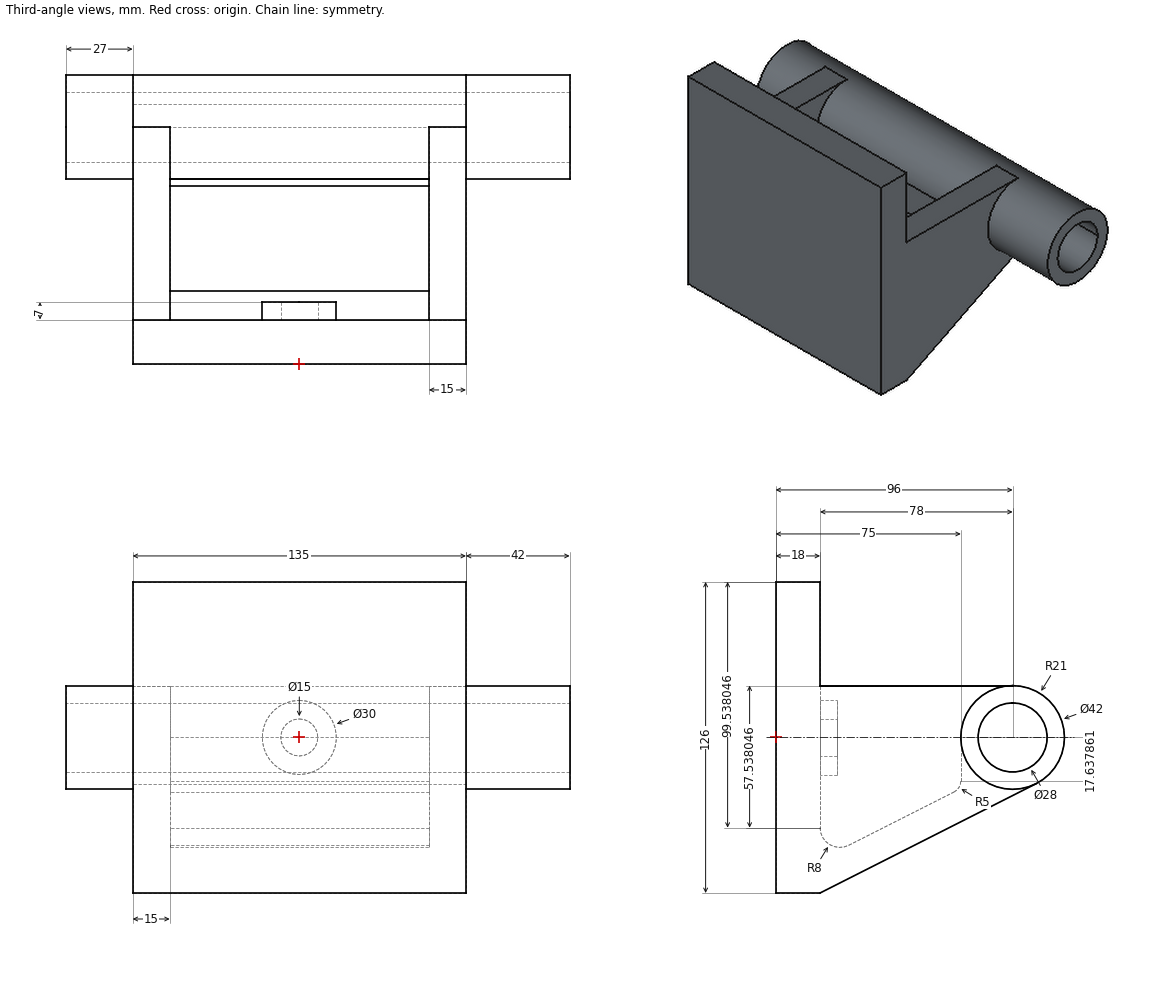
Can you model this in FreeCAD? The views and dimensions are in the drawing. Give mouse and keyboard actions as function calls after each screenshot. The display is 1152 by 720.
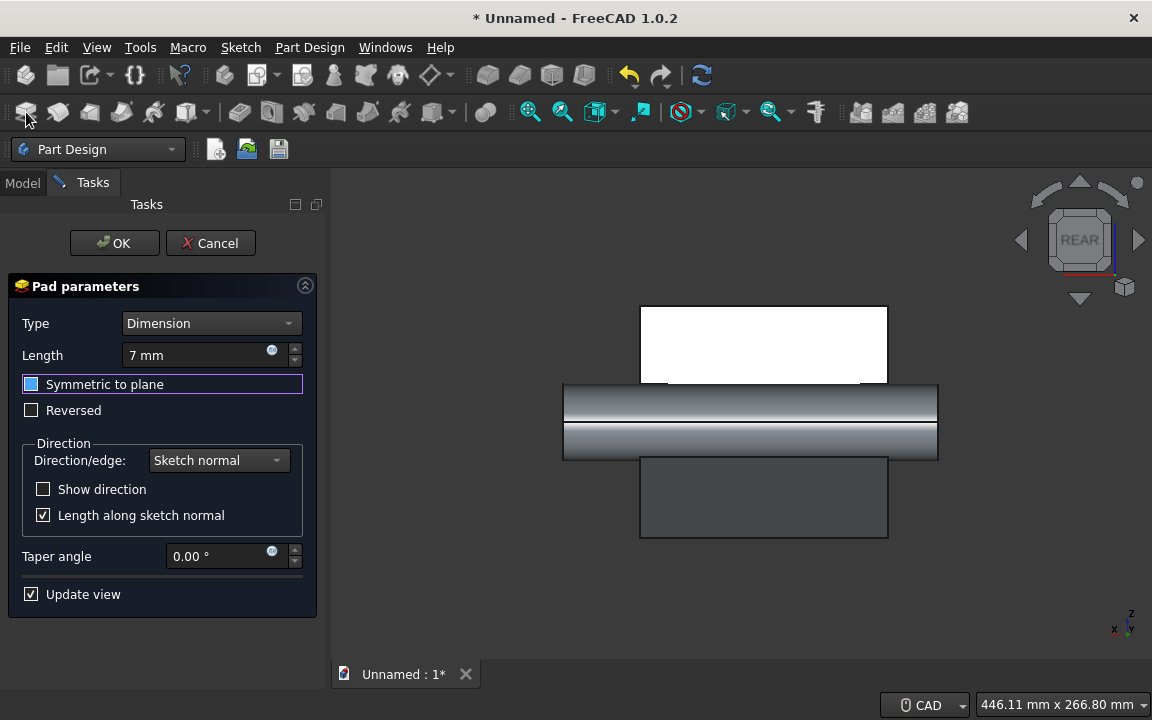
click(115, 243)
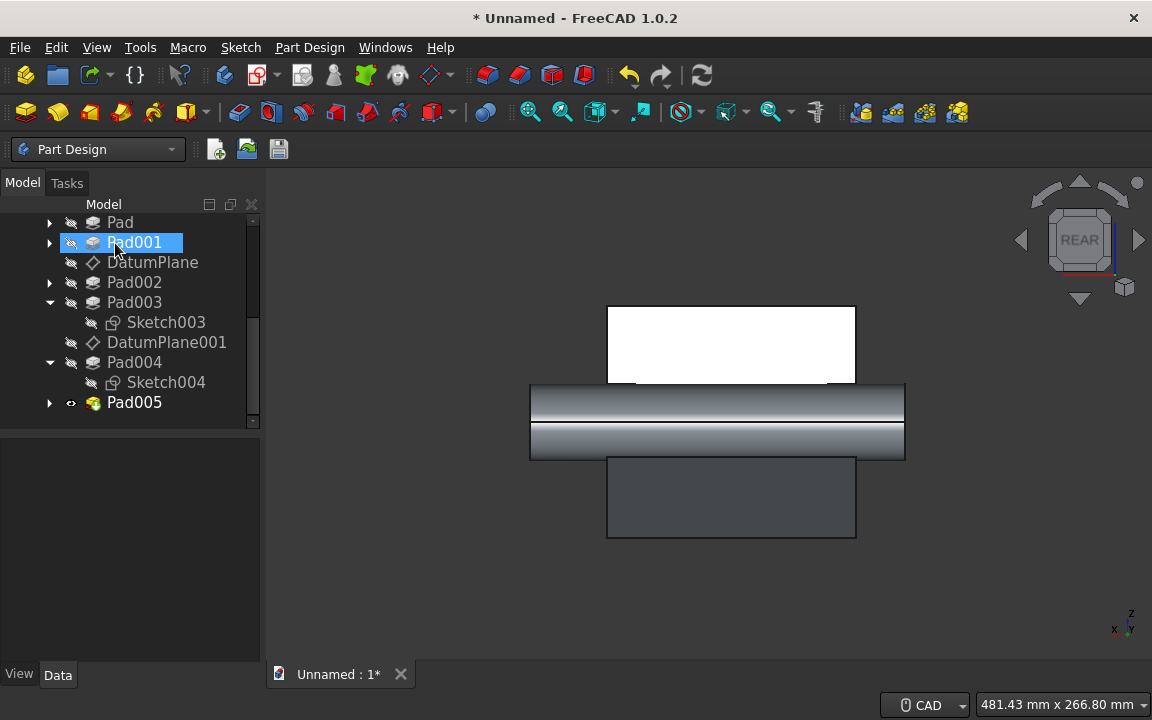
key(0)